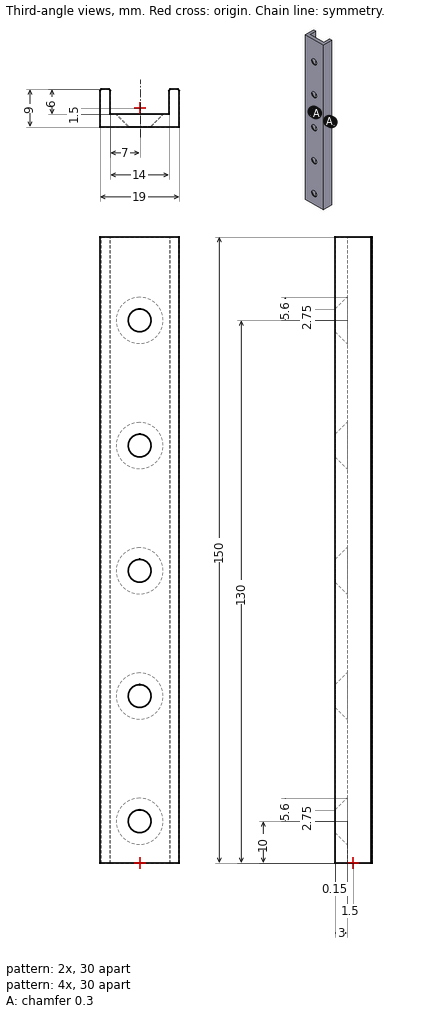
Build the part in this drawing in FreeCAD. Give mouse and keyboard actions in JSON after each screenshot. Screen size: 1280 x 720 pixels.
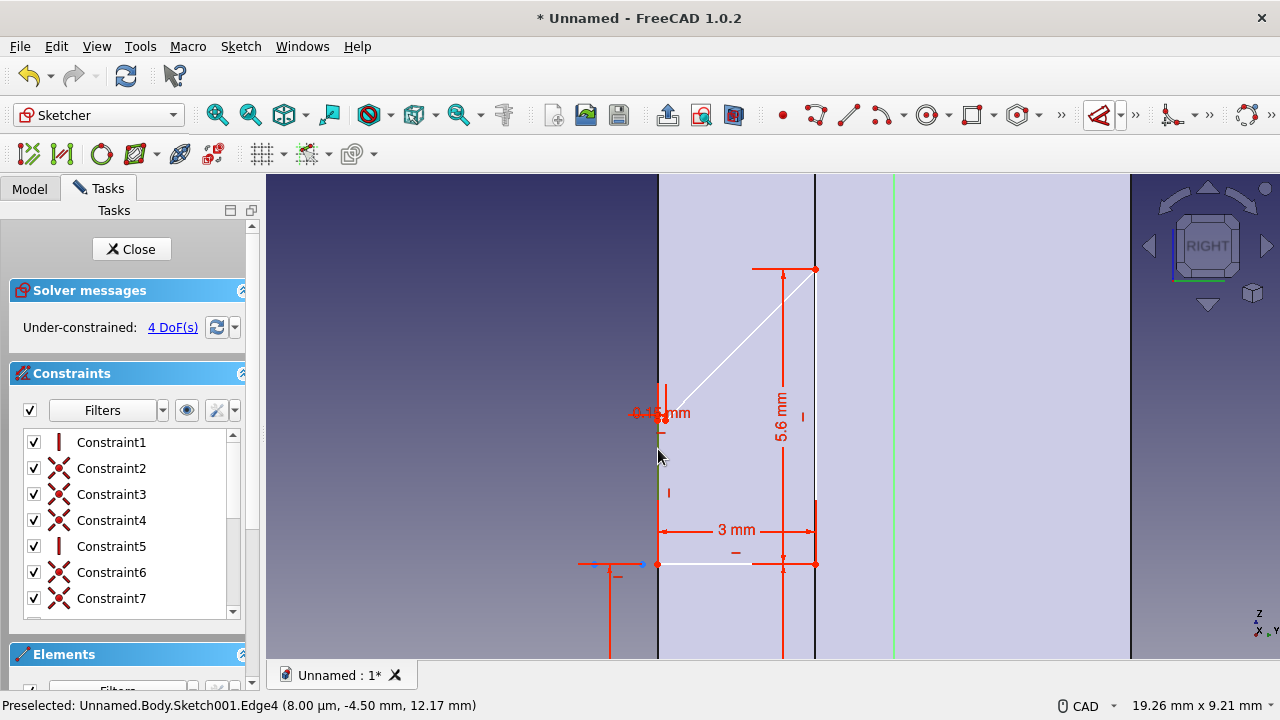
{"action": "key", "text": "i"}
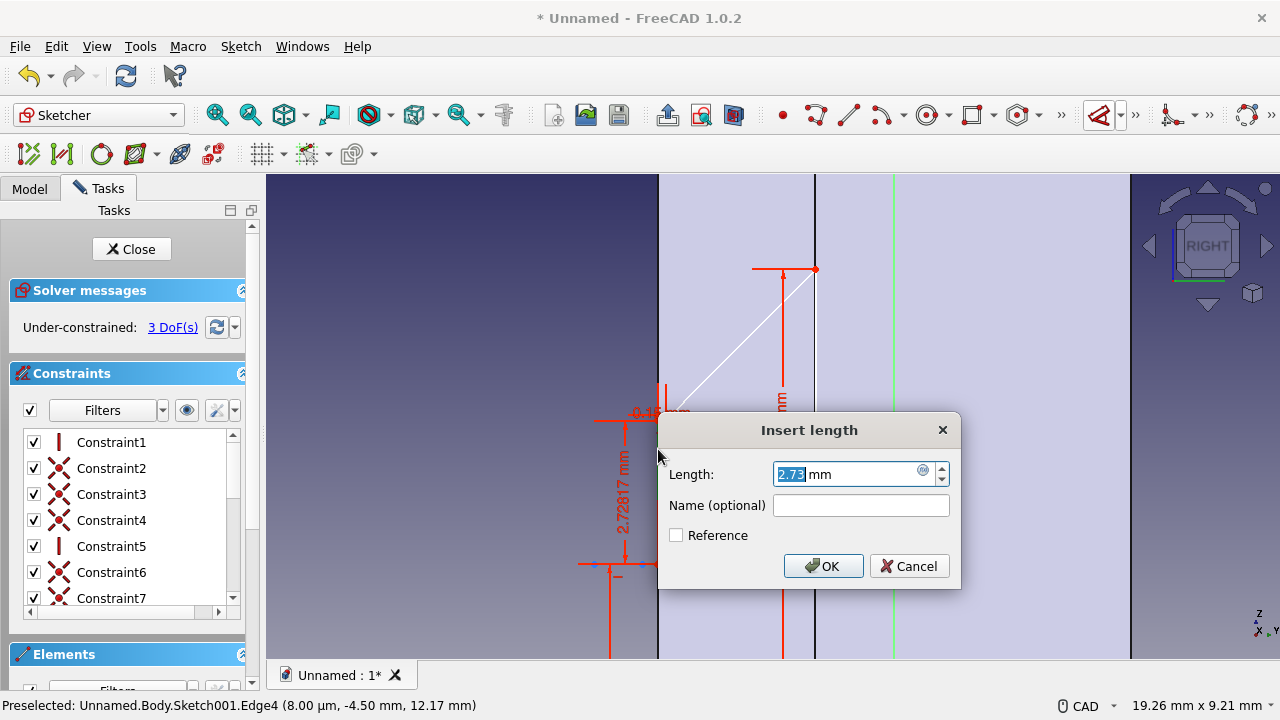
{"action": "type", "text": "2.75"}
{"action": "key", "text": "Return"}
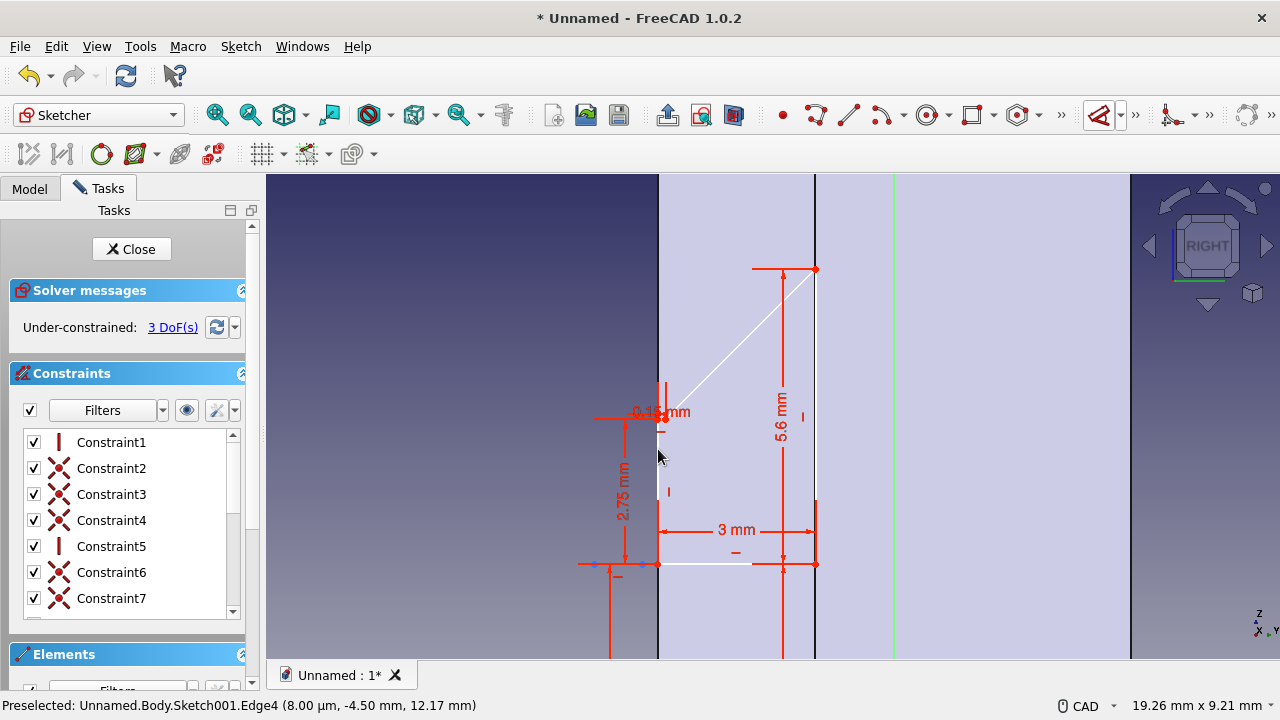
{"action": "left_click", "coordinate": [816, 564]}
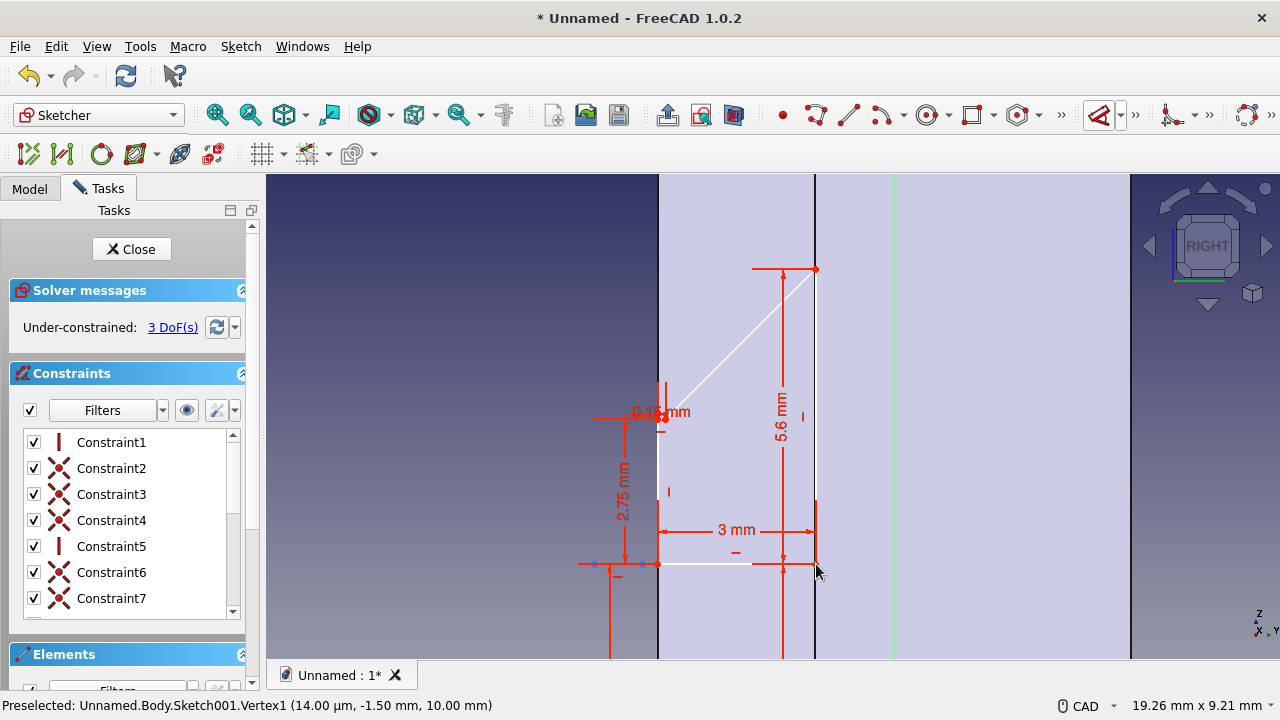
{"action": "key", "text": "l"}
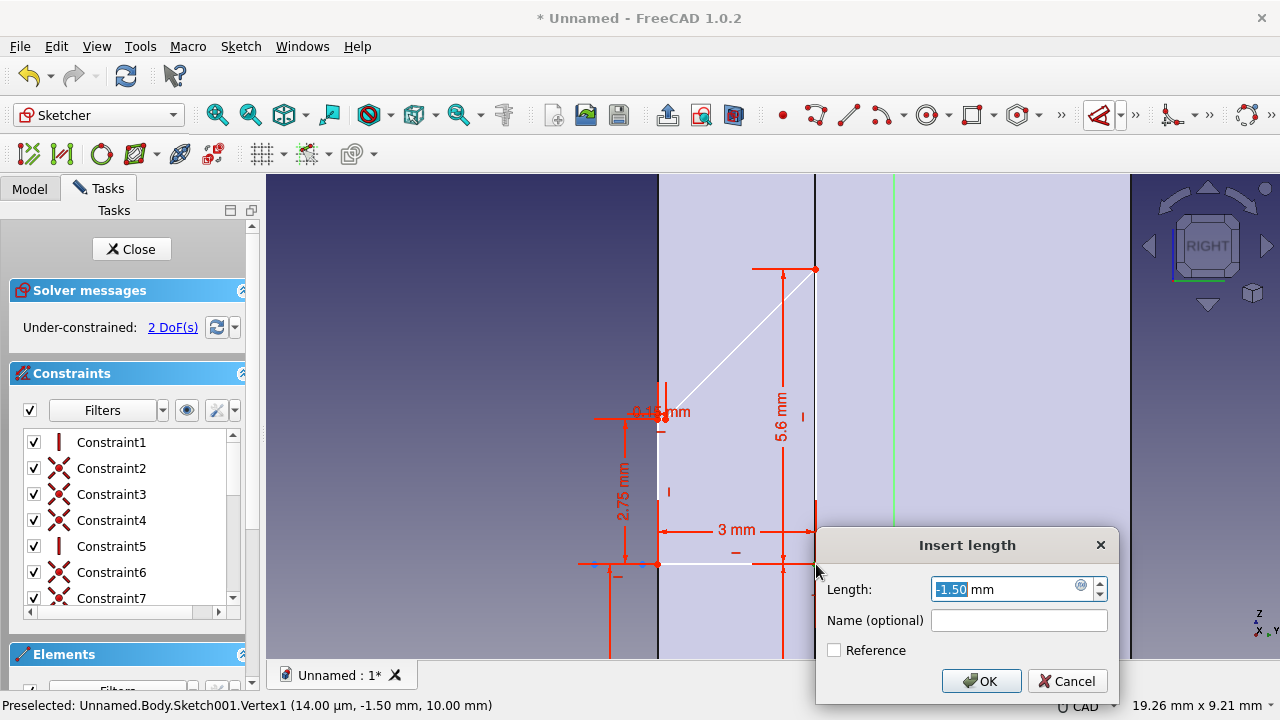
{"action": "type", "text": "-1.5"}
{"action": "key", "text": "Return"}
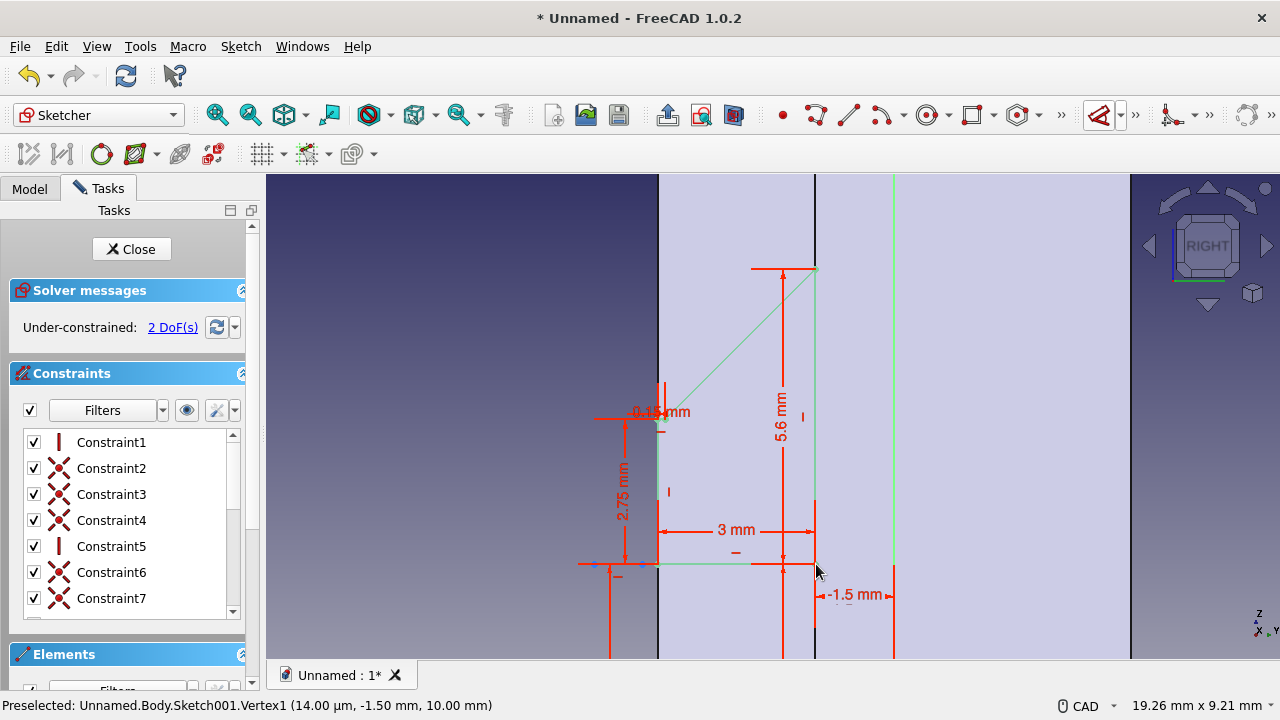
{"action": "left_click", "coordinate": [132, 249]}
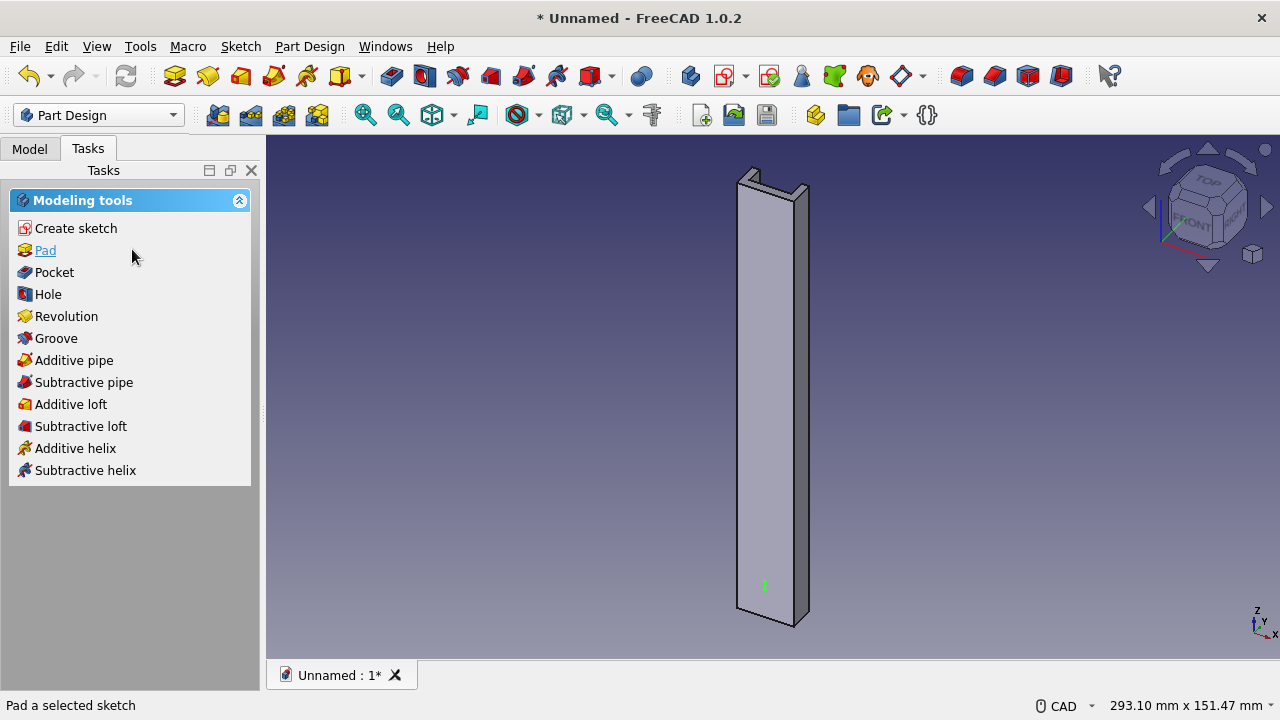
{"action": "left_click", "coordinate": [458, 76]}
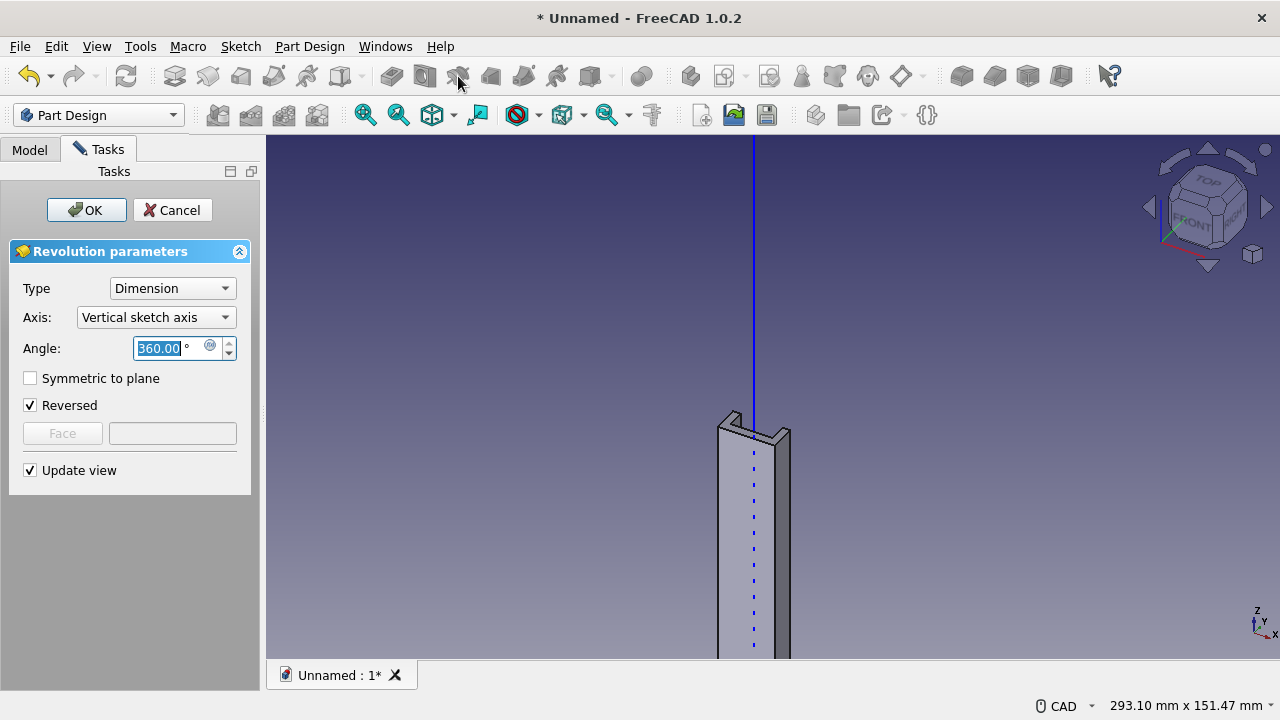
{"action": "left_click", "coordinate": [157, 318]}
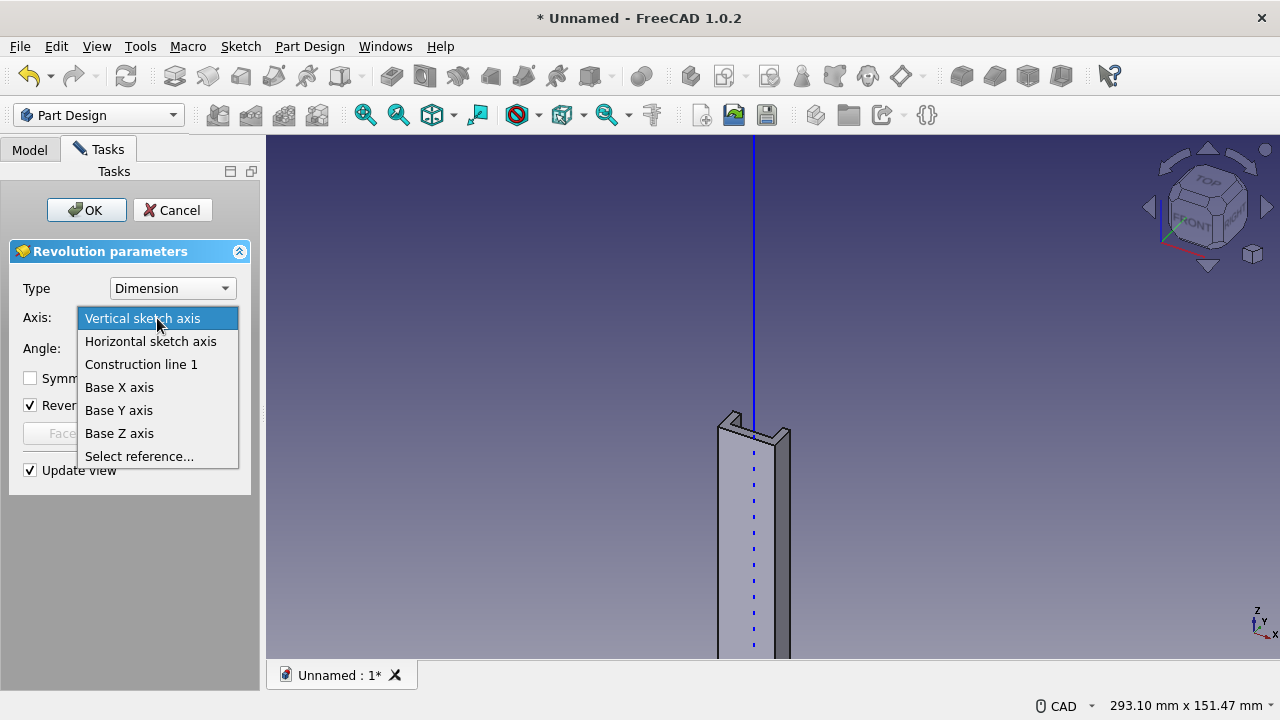
{"action": "left_click", "coordinate": [156, 364]}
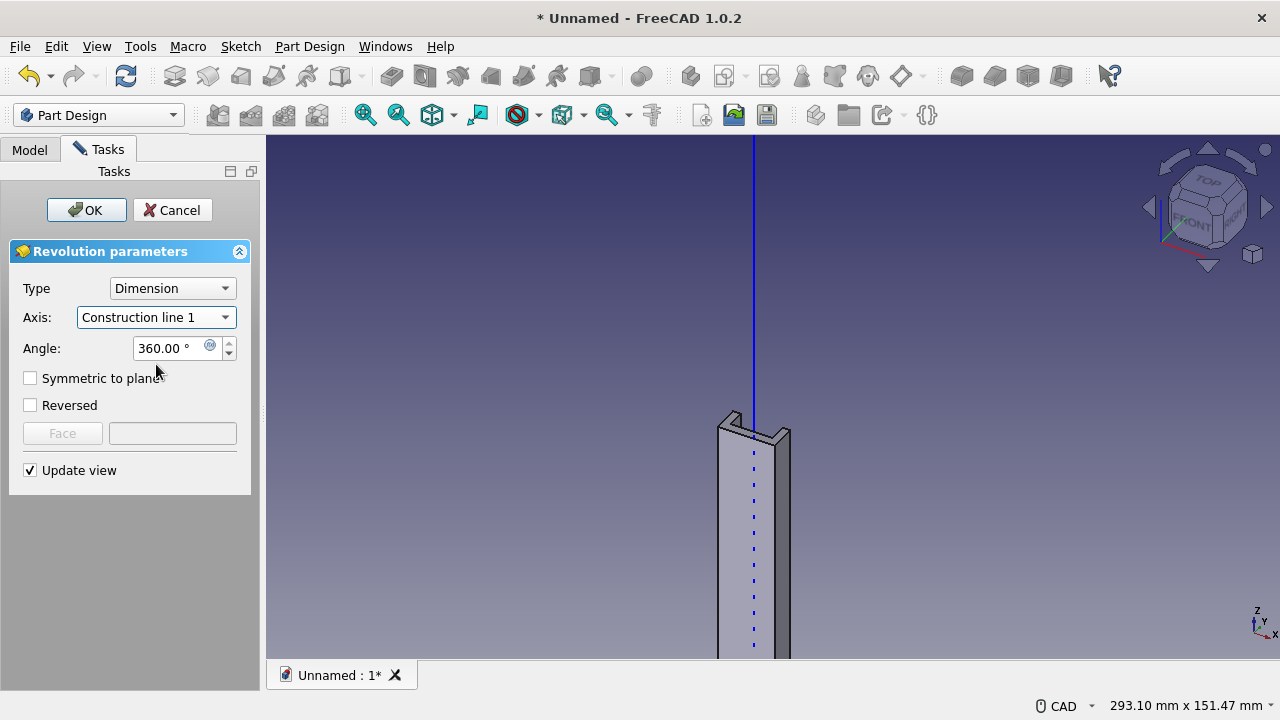
{"action": "left_click", "coordinate": [87, 210]}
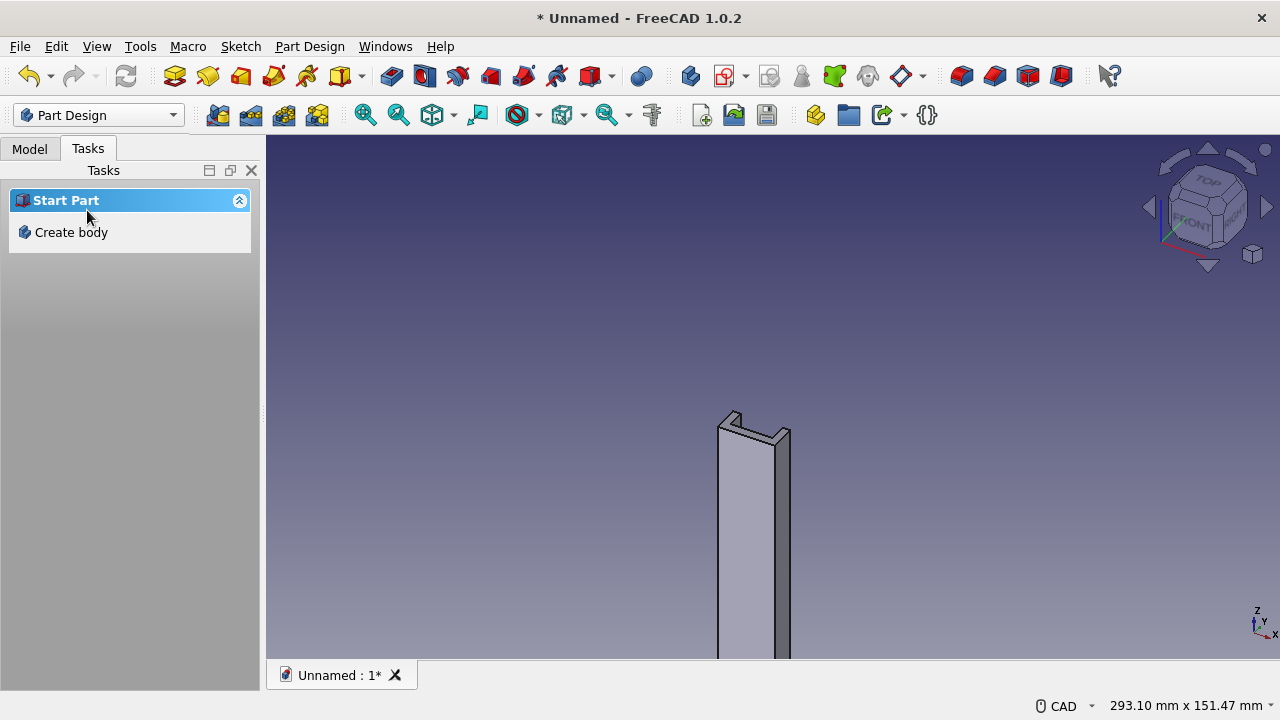
{"action": "left_click", "coordinate": [366, 116]}